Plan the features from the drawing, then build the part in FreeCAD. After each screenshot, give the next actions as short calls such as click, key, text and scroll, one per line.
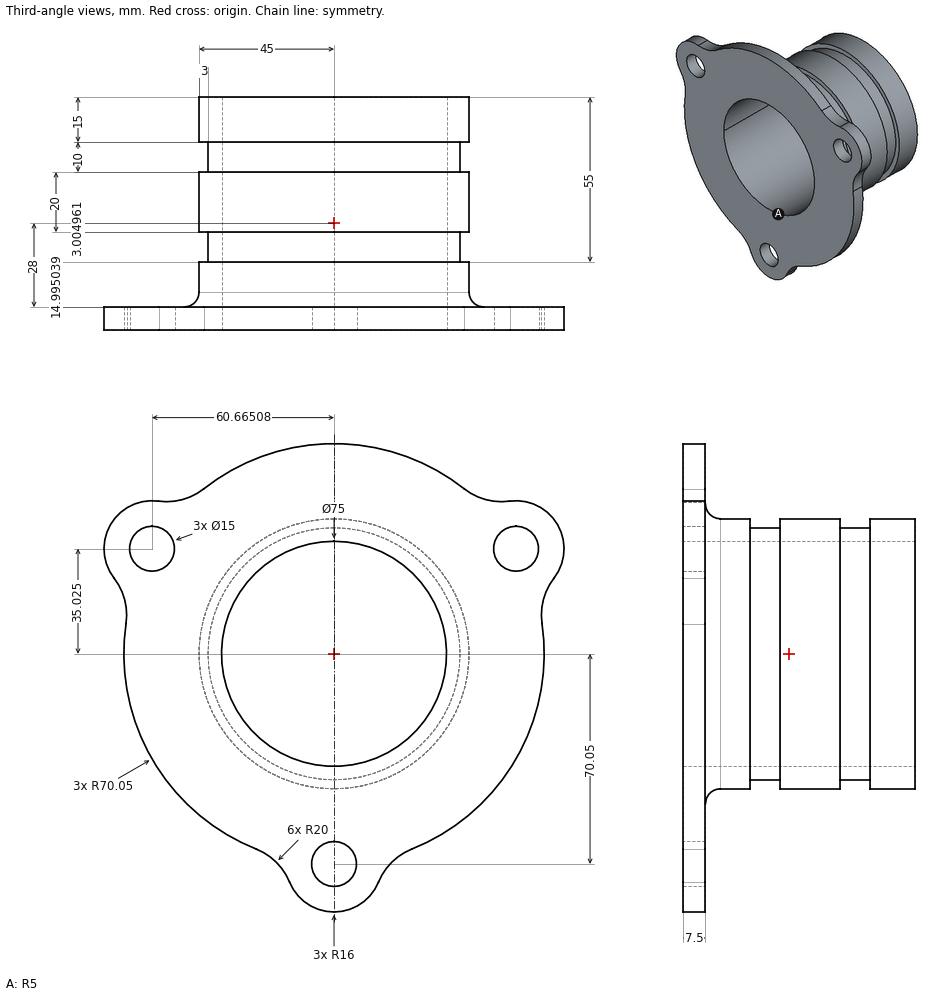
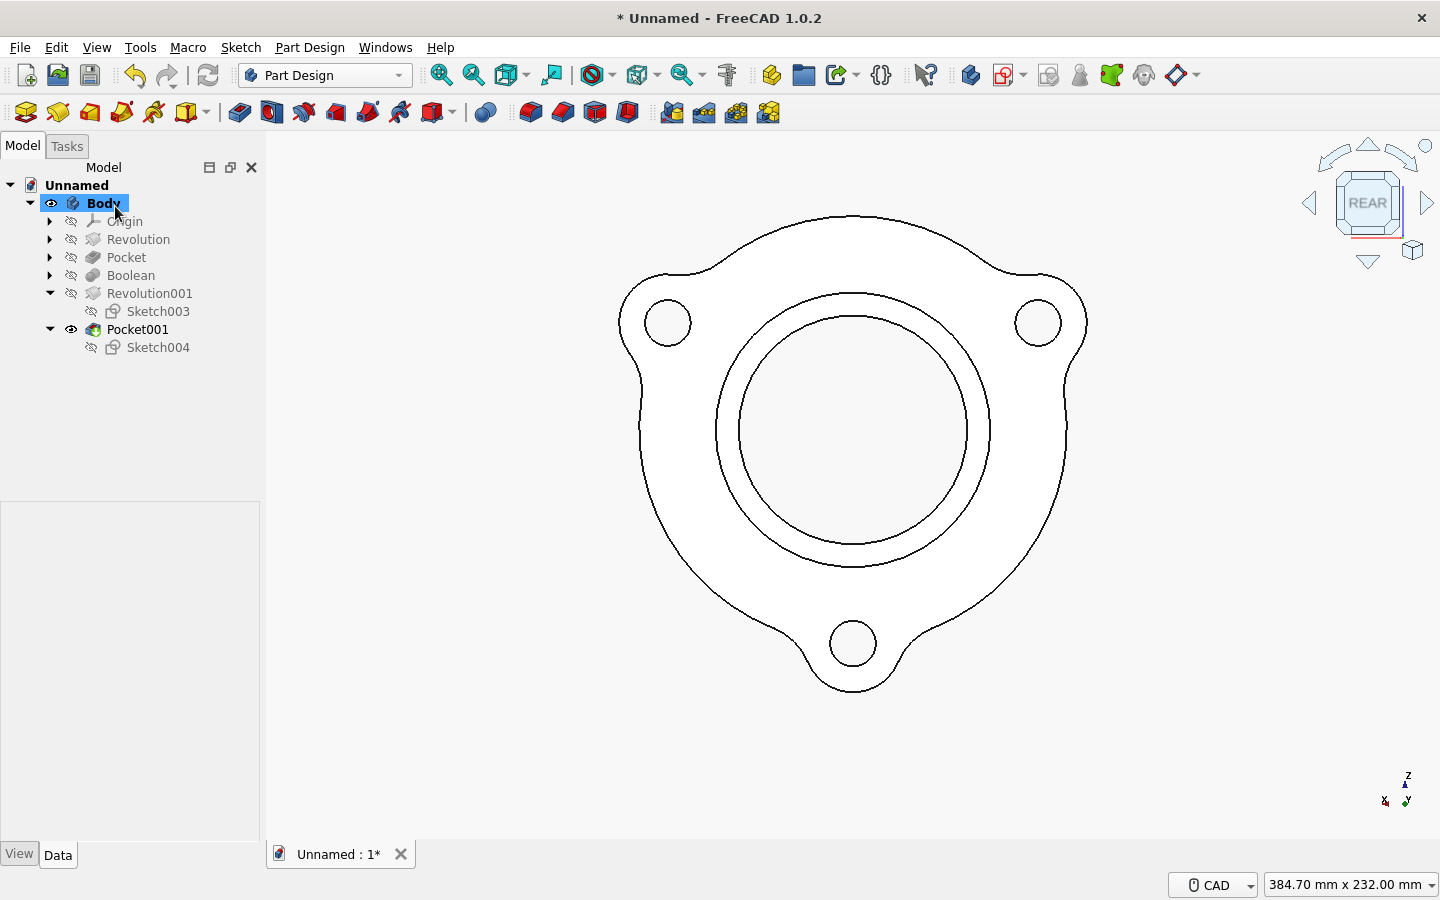
key(0)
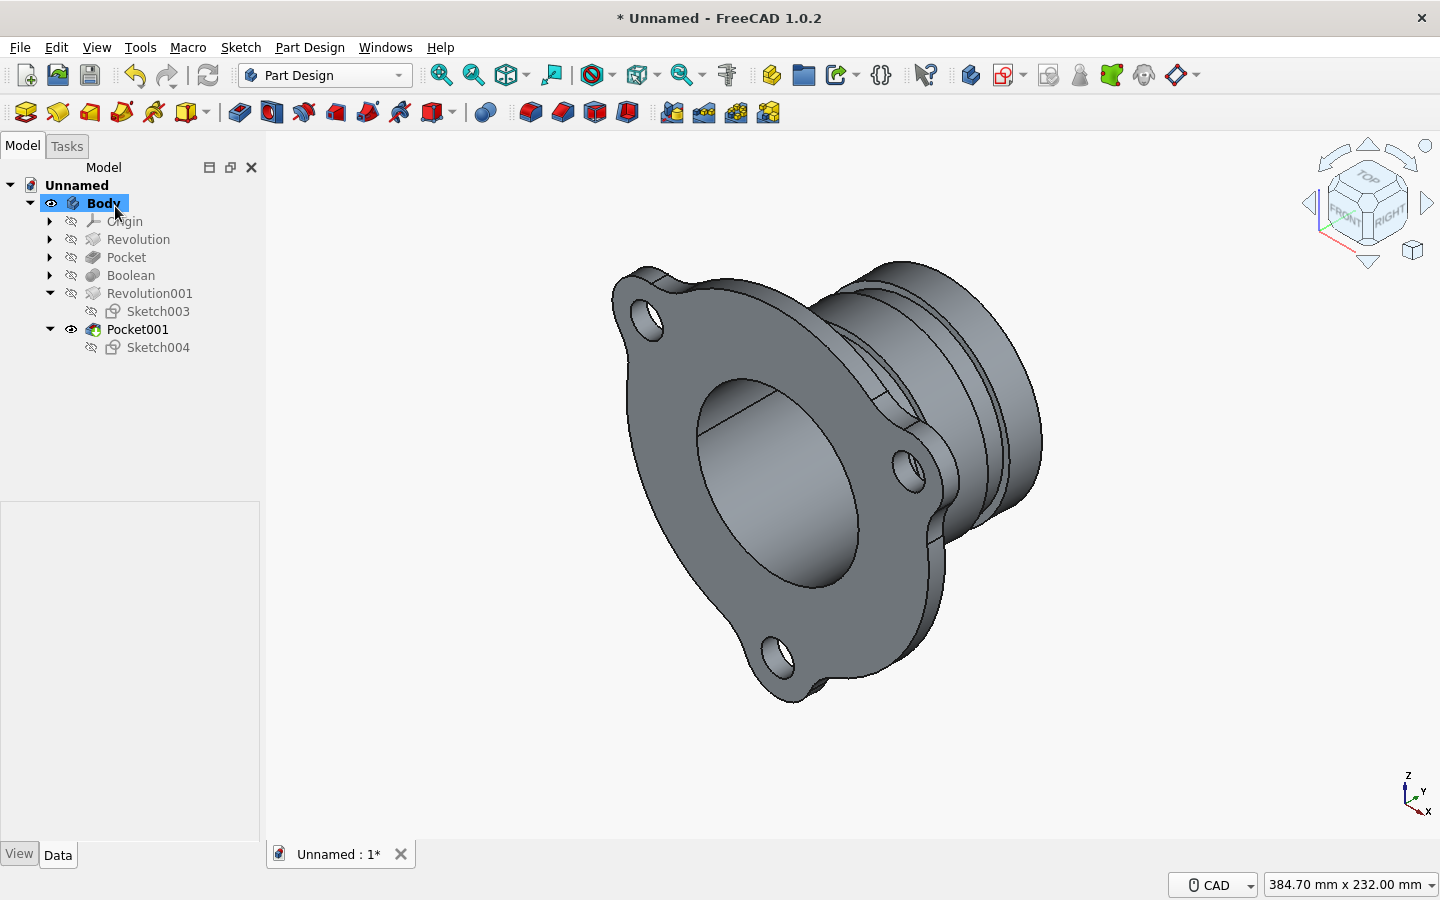
key(v)
key(f)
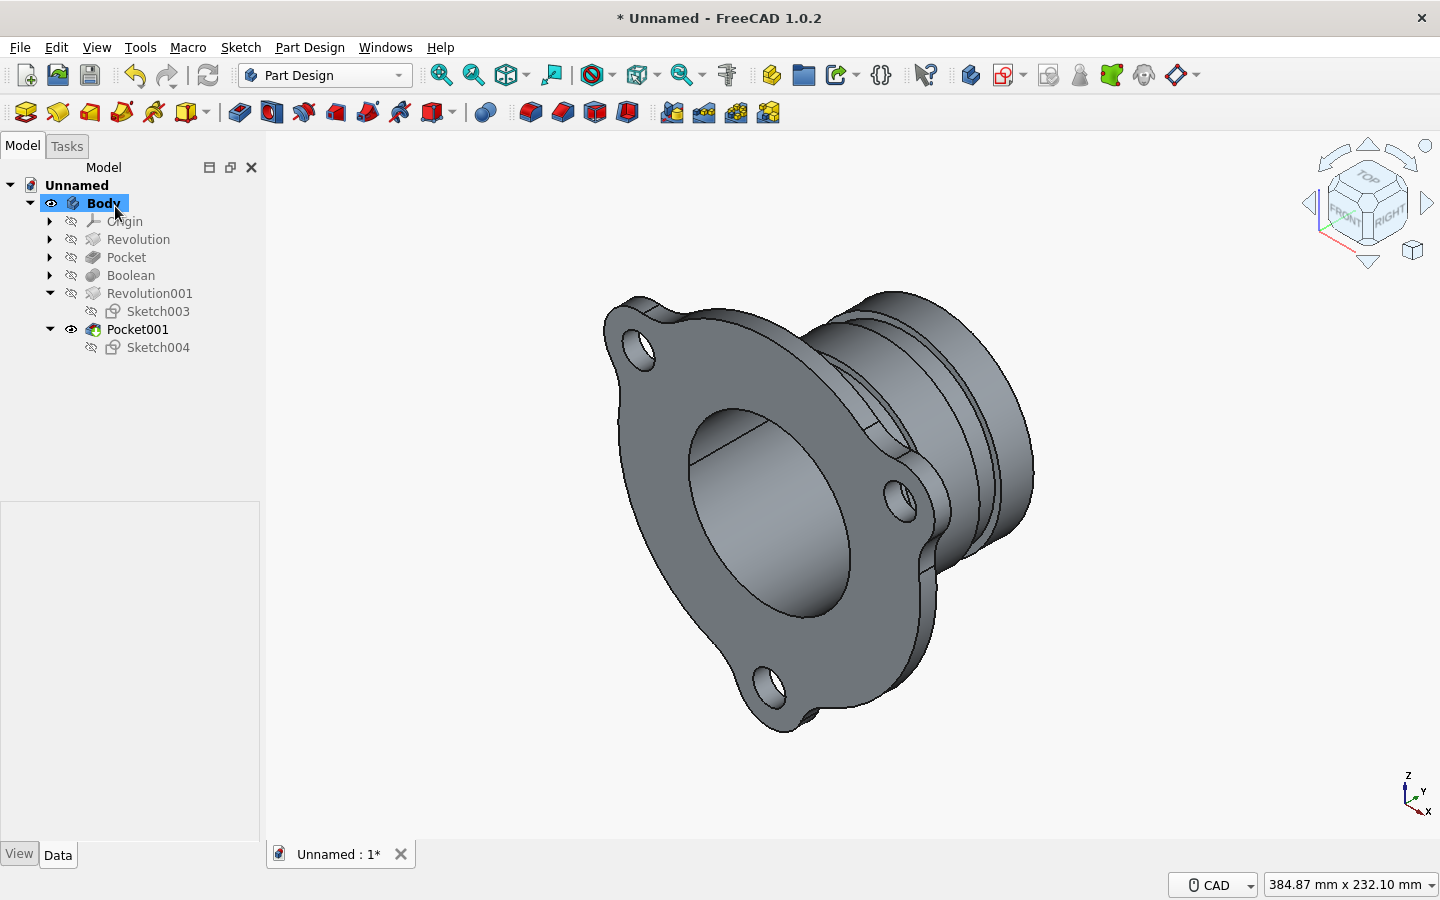
key(2)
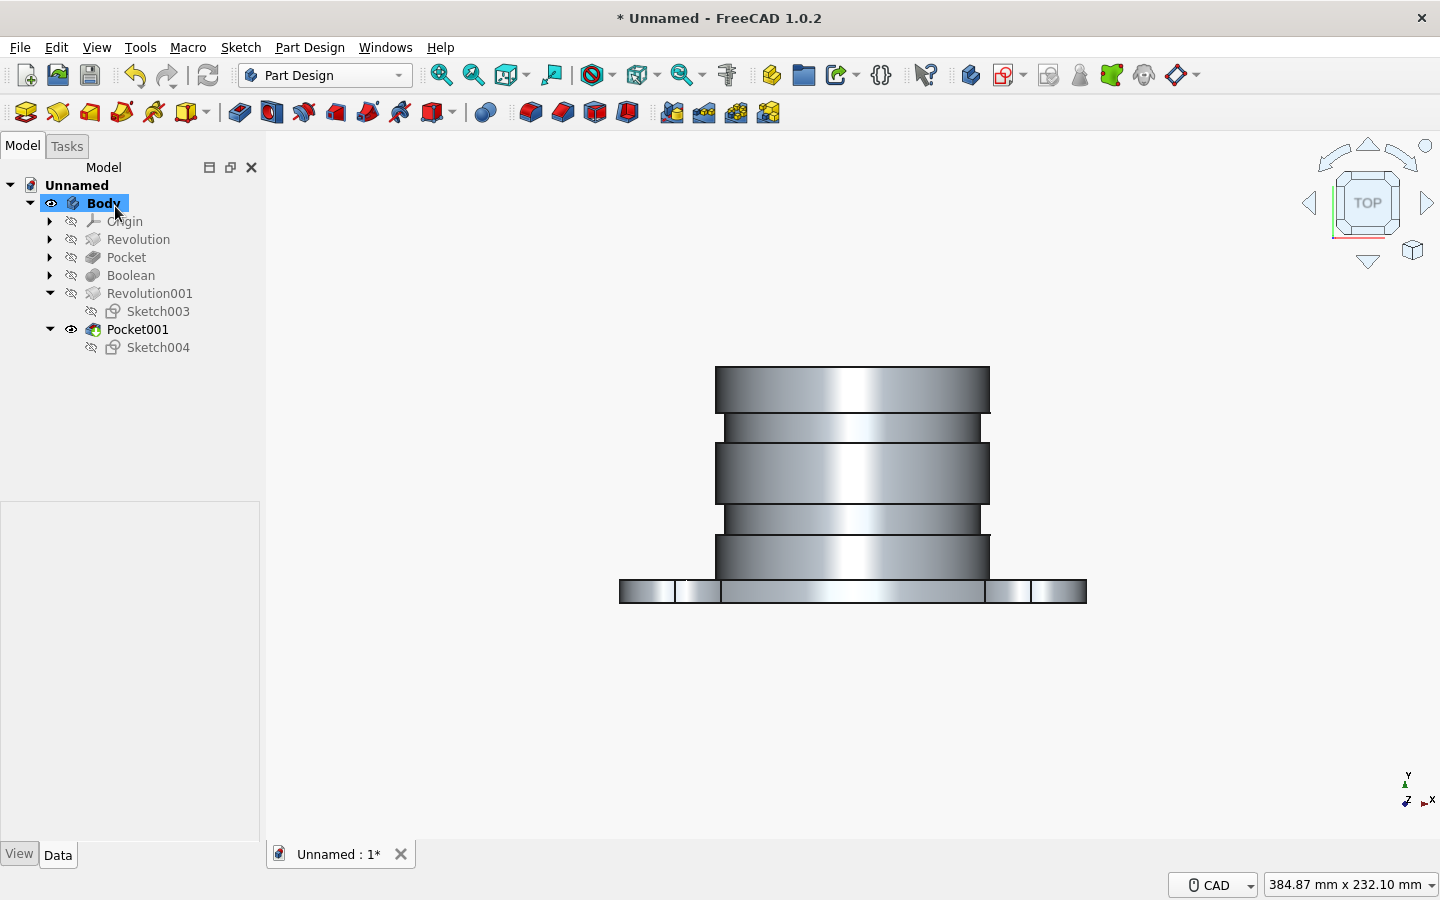
key(v)
key(f)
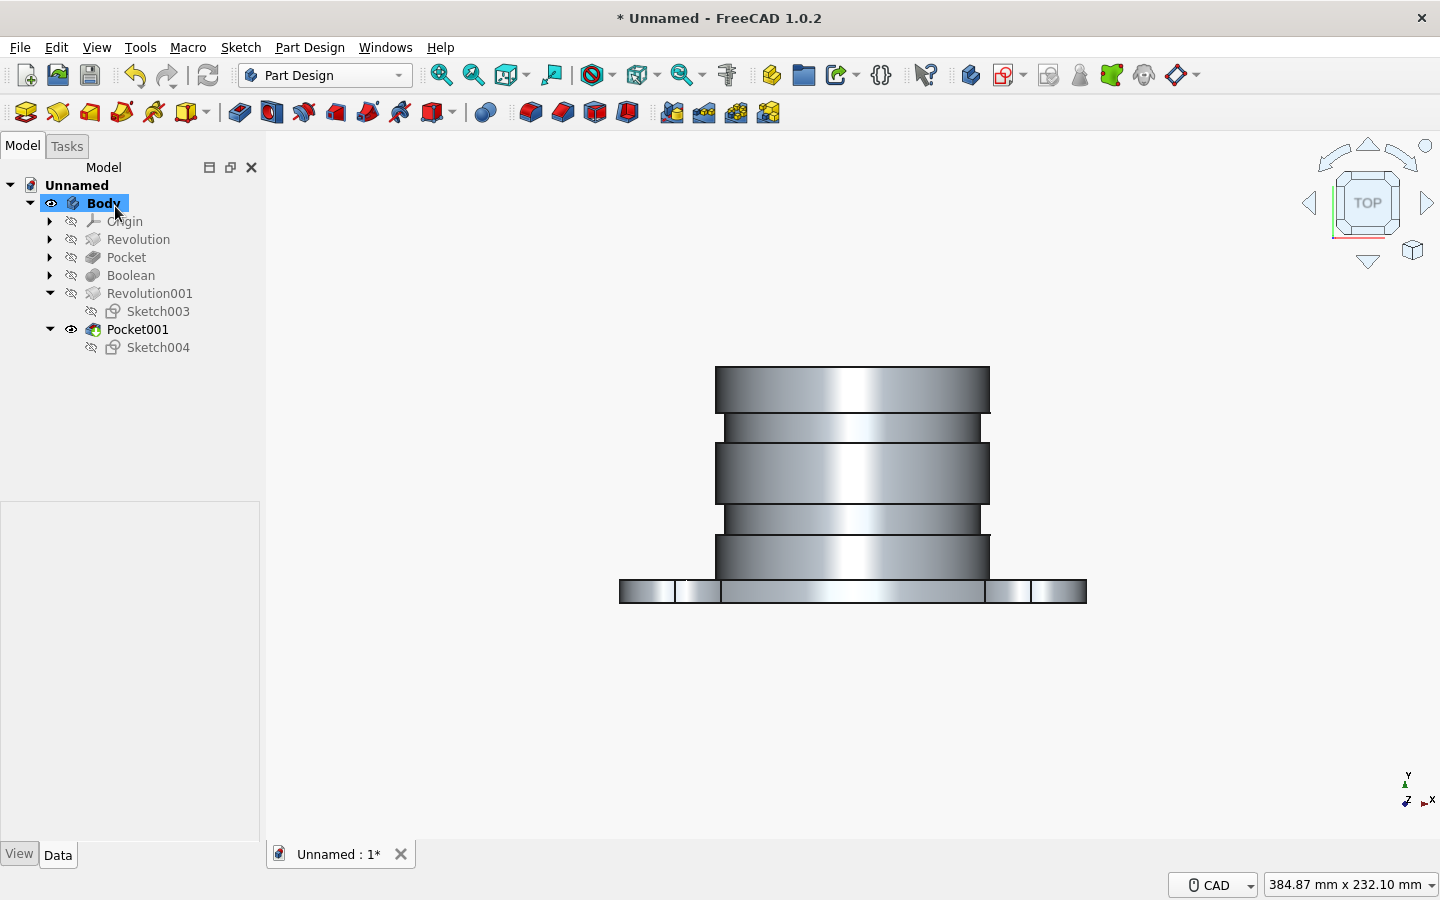
key(1)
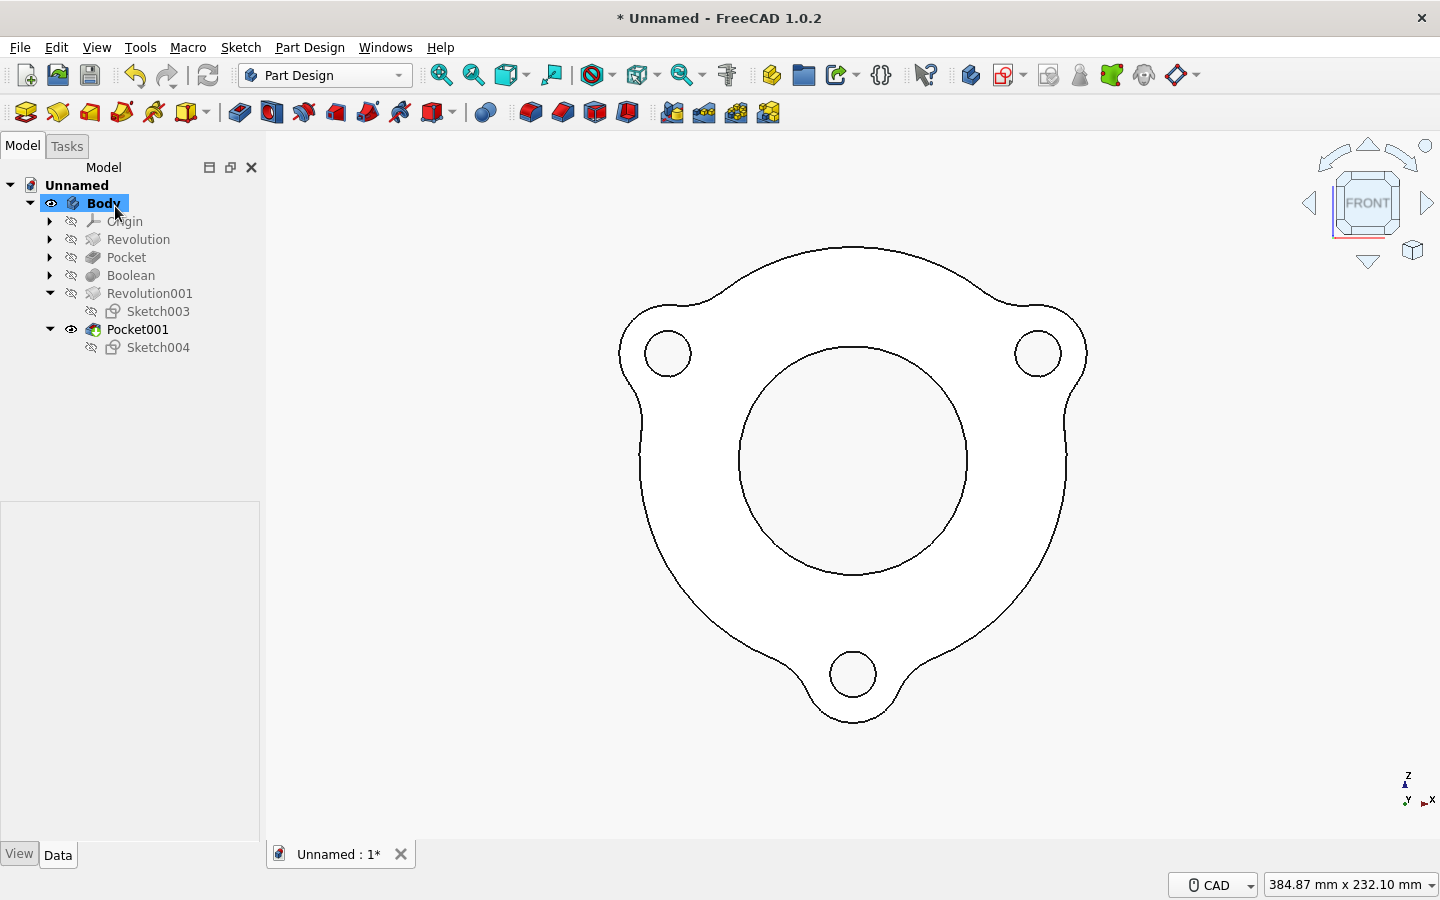
key(3)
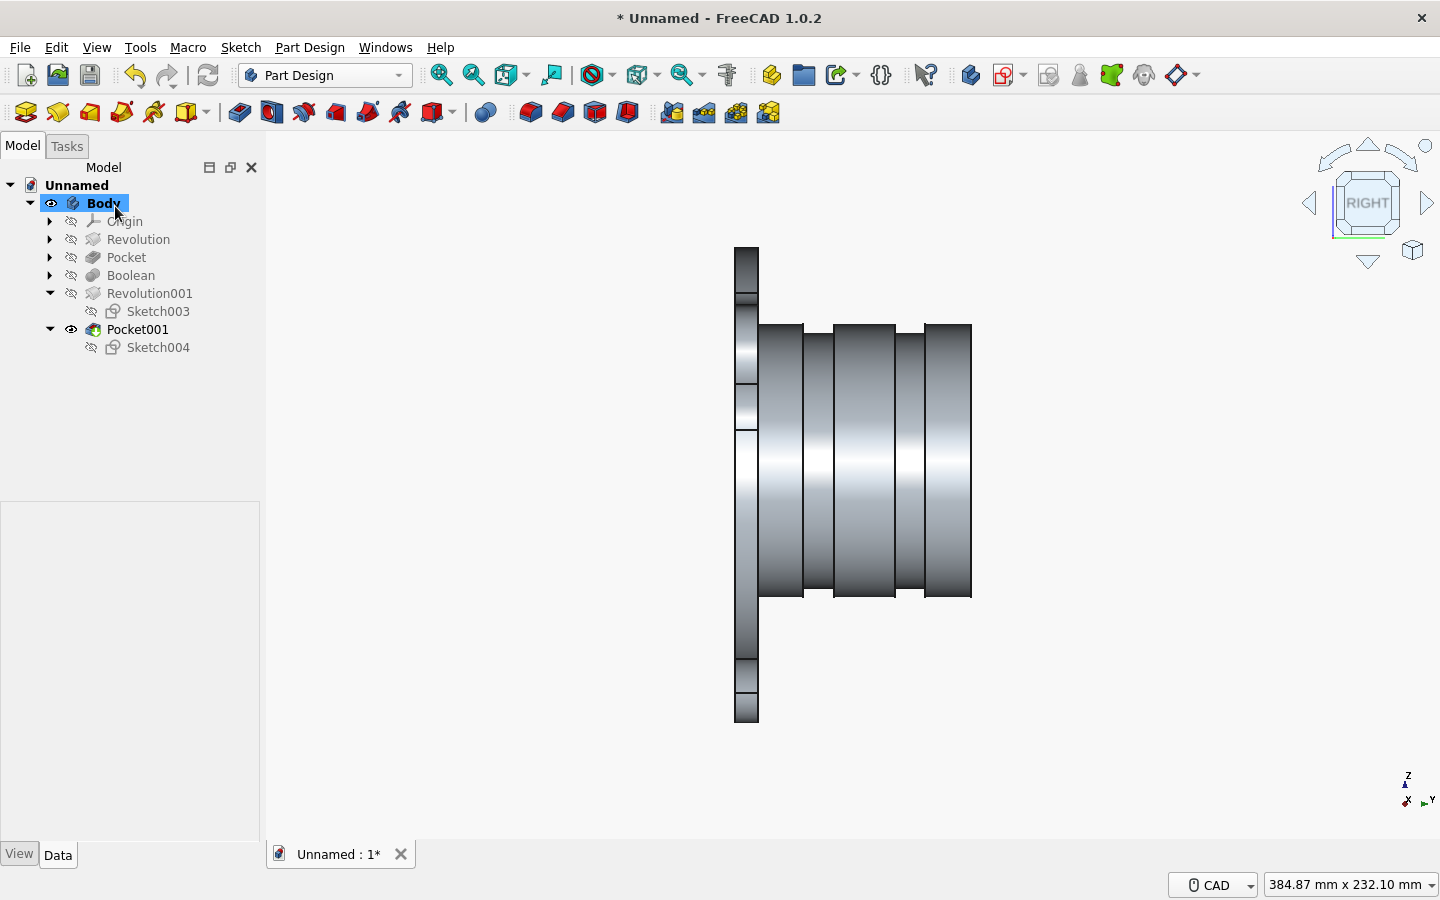
key(5)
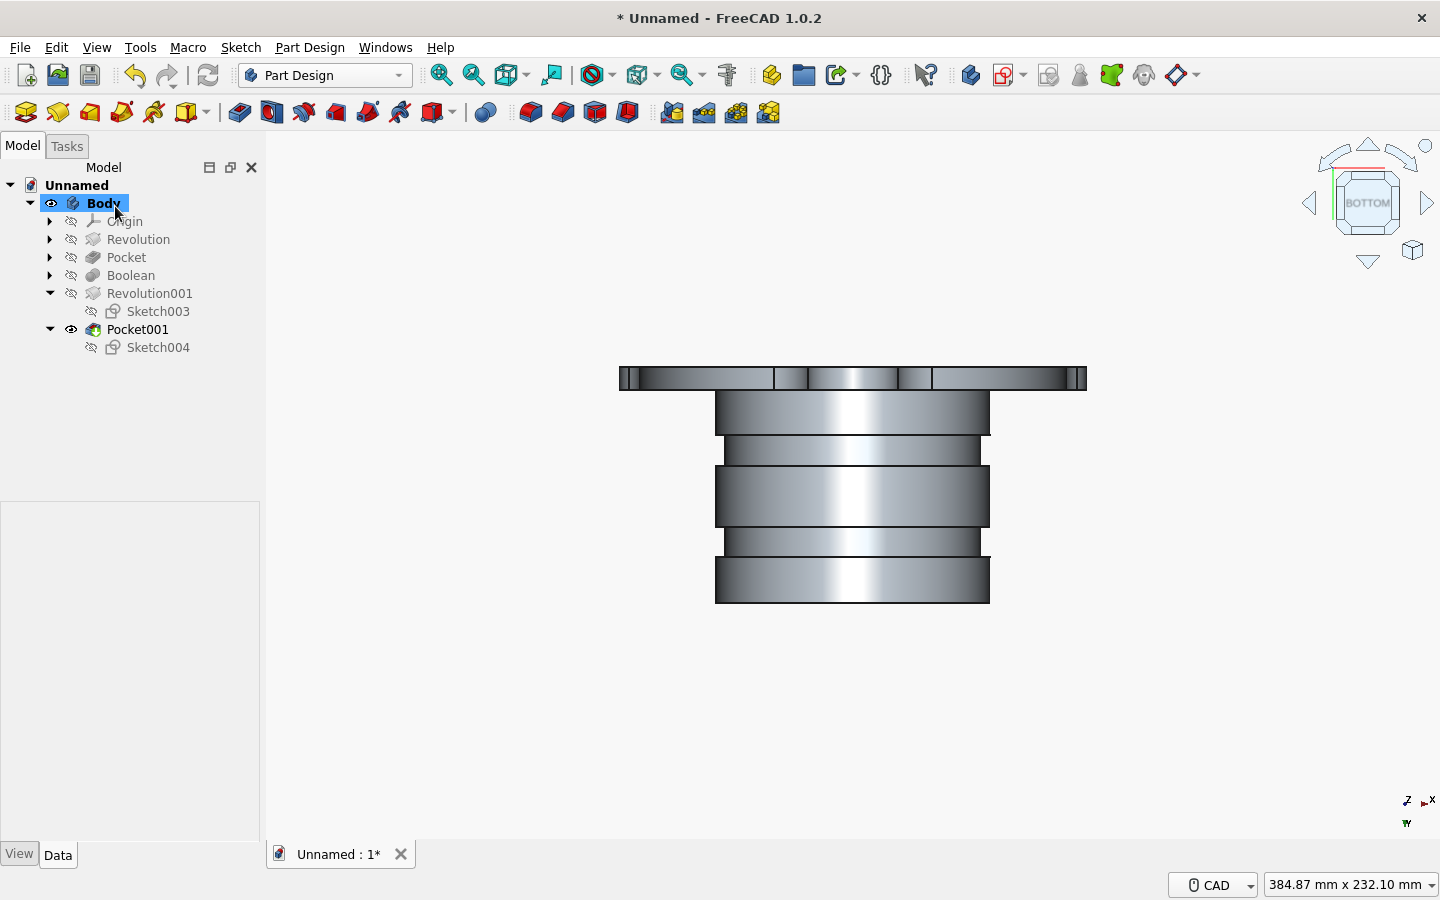
key(v)
key(f)